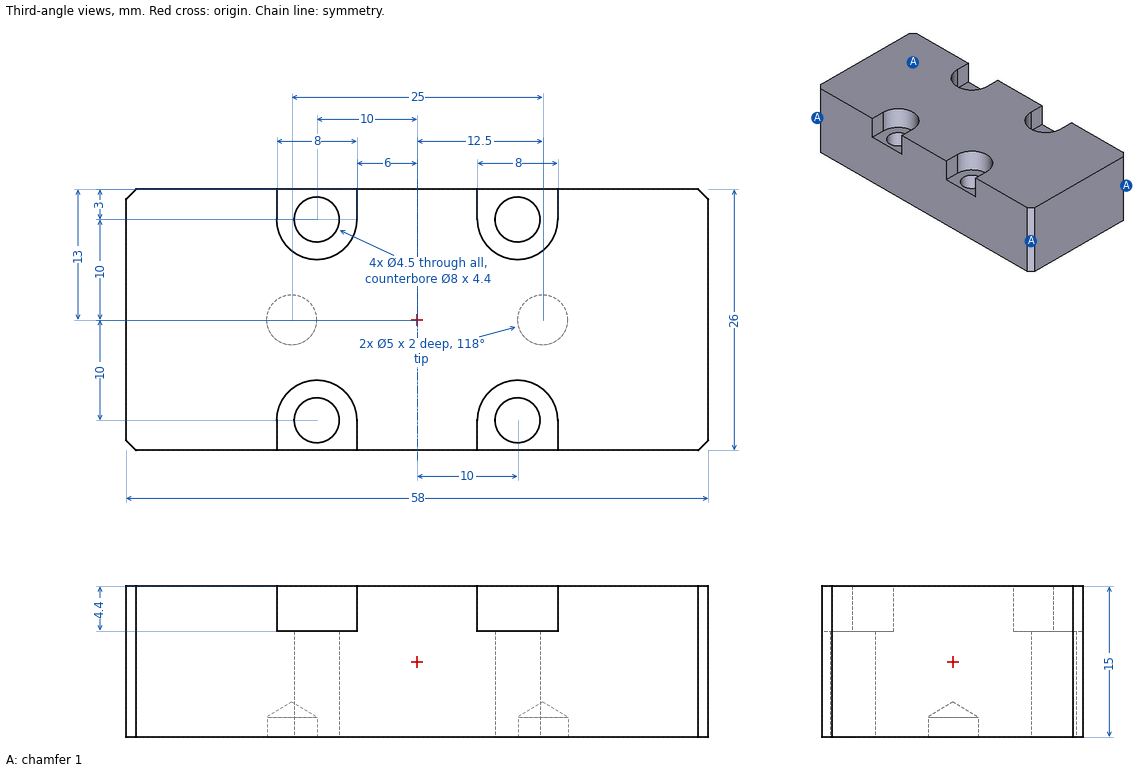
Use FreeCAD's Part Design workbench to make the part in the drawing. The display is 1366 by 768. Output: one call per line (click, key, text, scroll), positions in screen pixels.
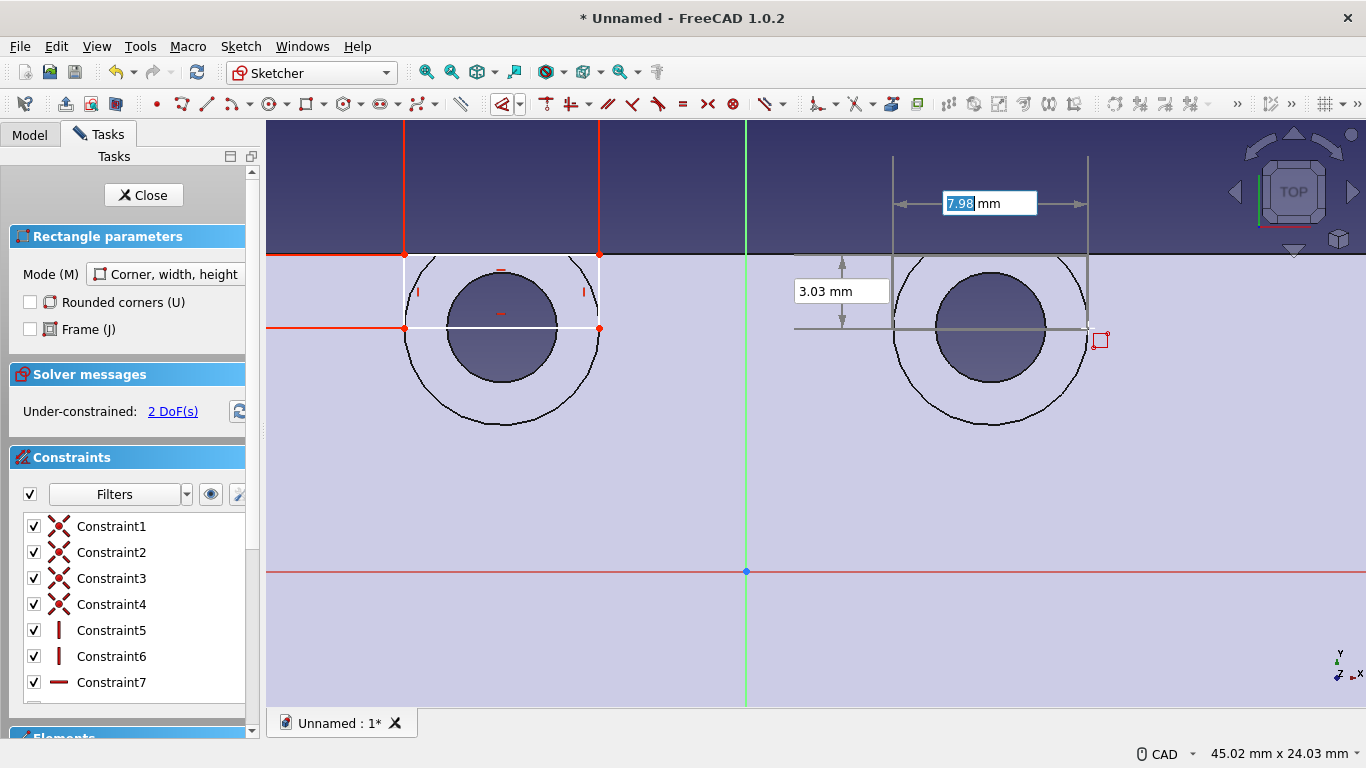
text(8)
key(Tab)
text(3)
key(Return)
key(Escape)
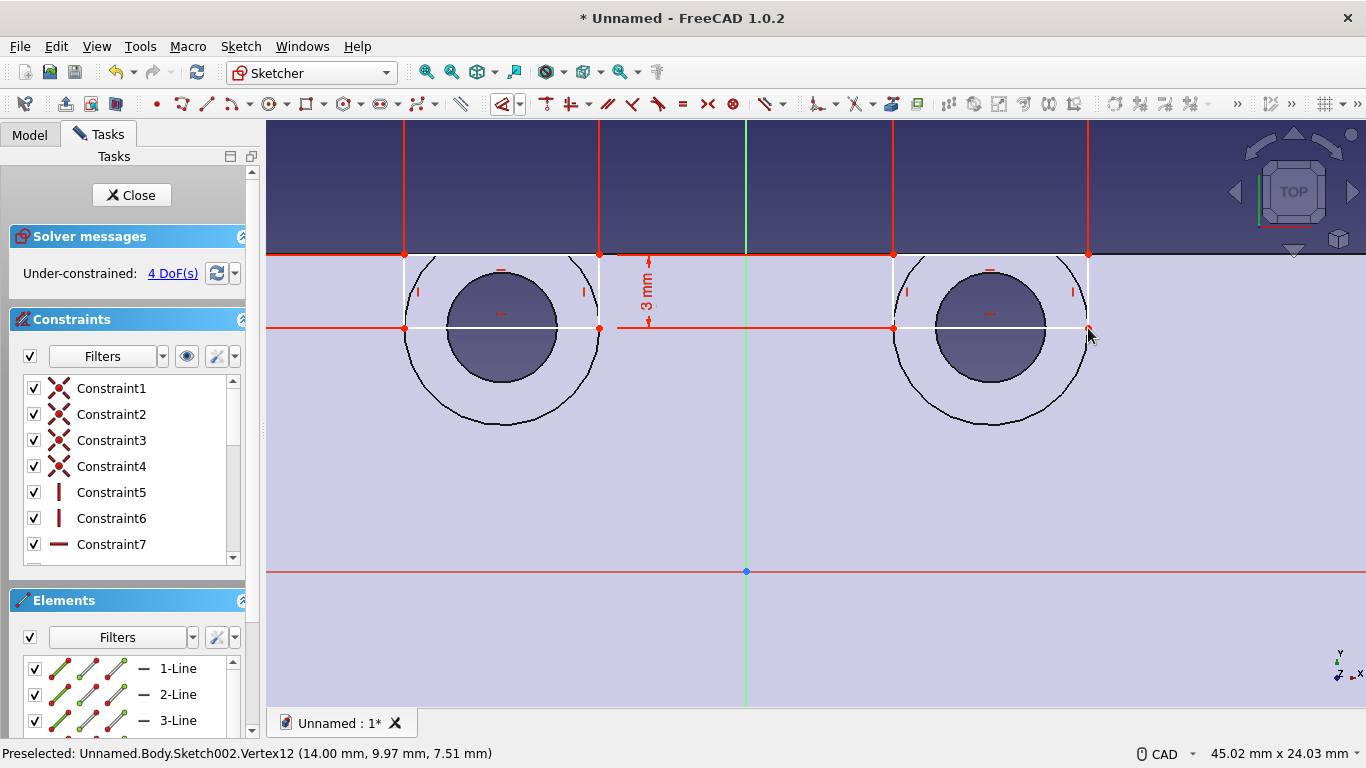
click(599, 255)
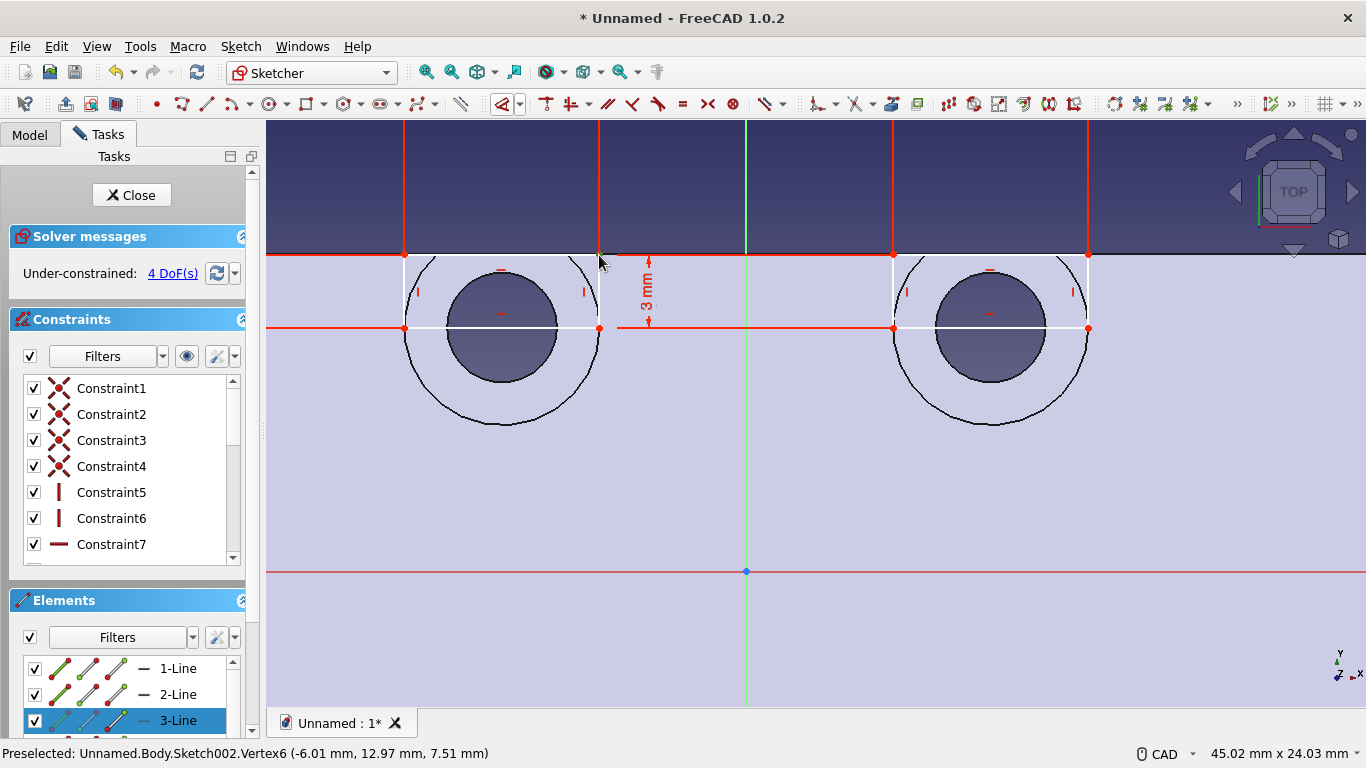
click(893, 255)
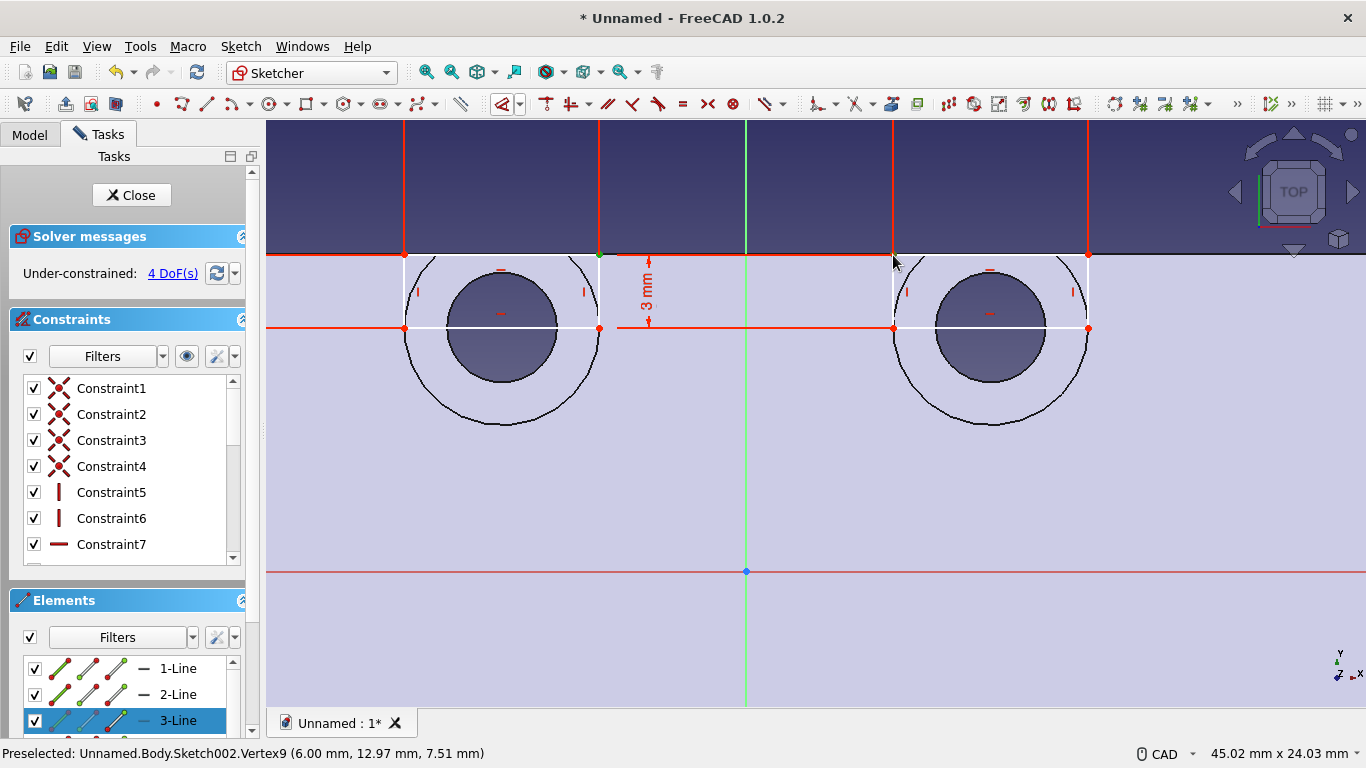
click(746, 641)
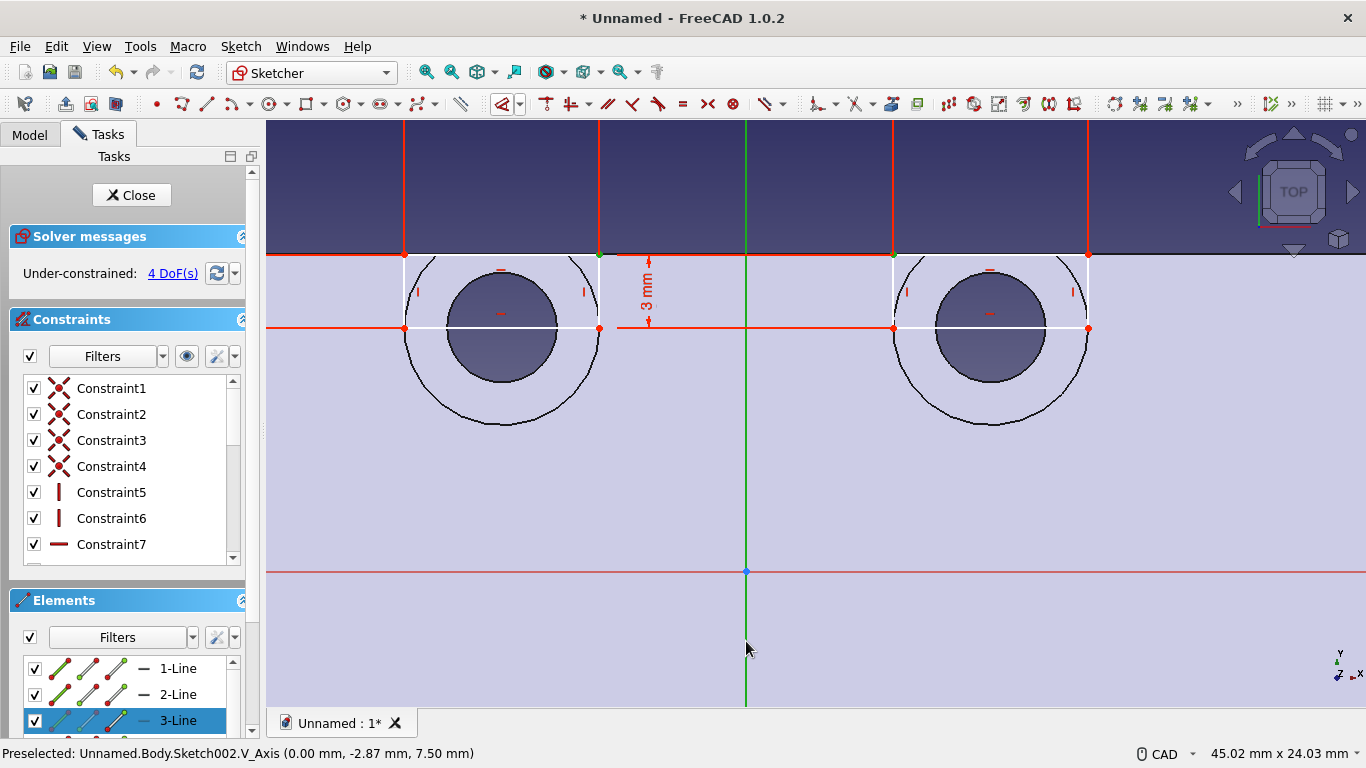
key(s)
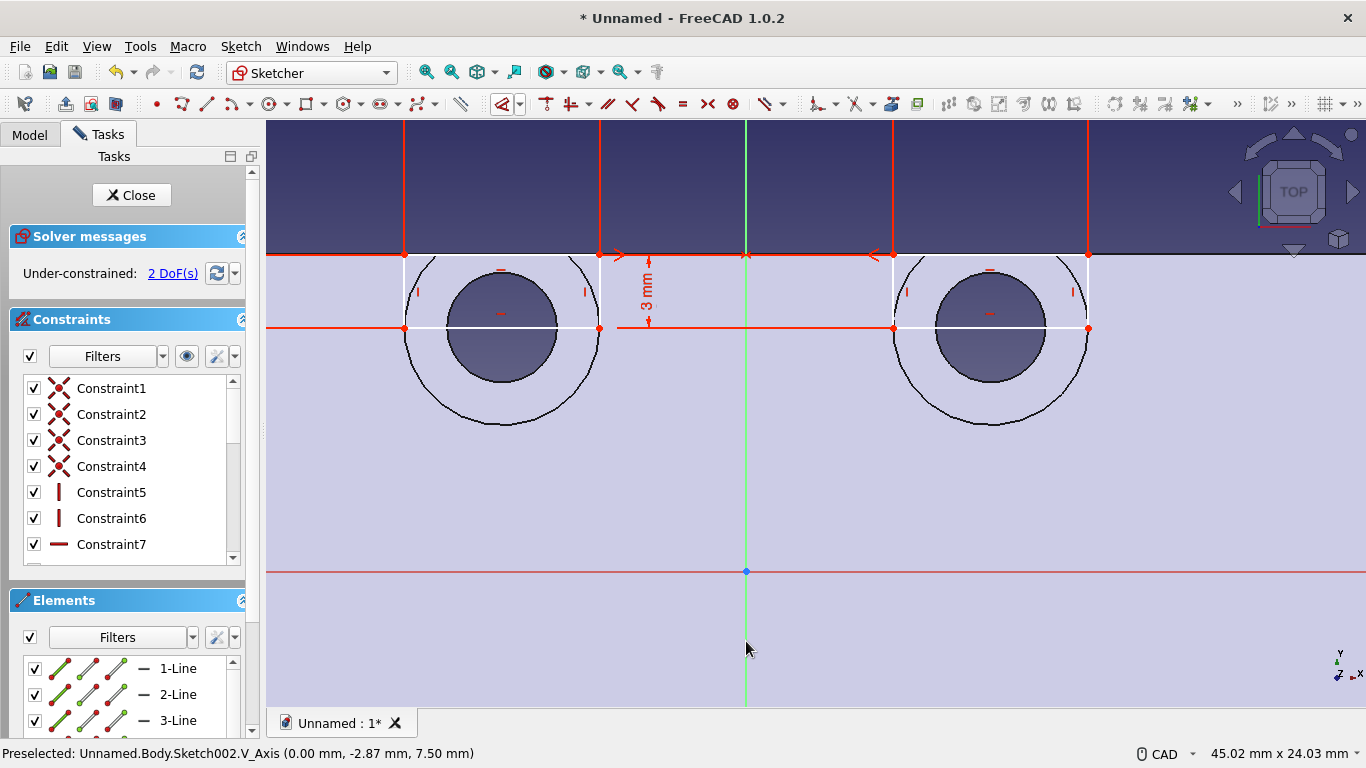
click(600, 328)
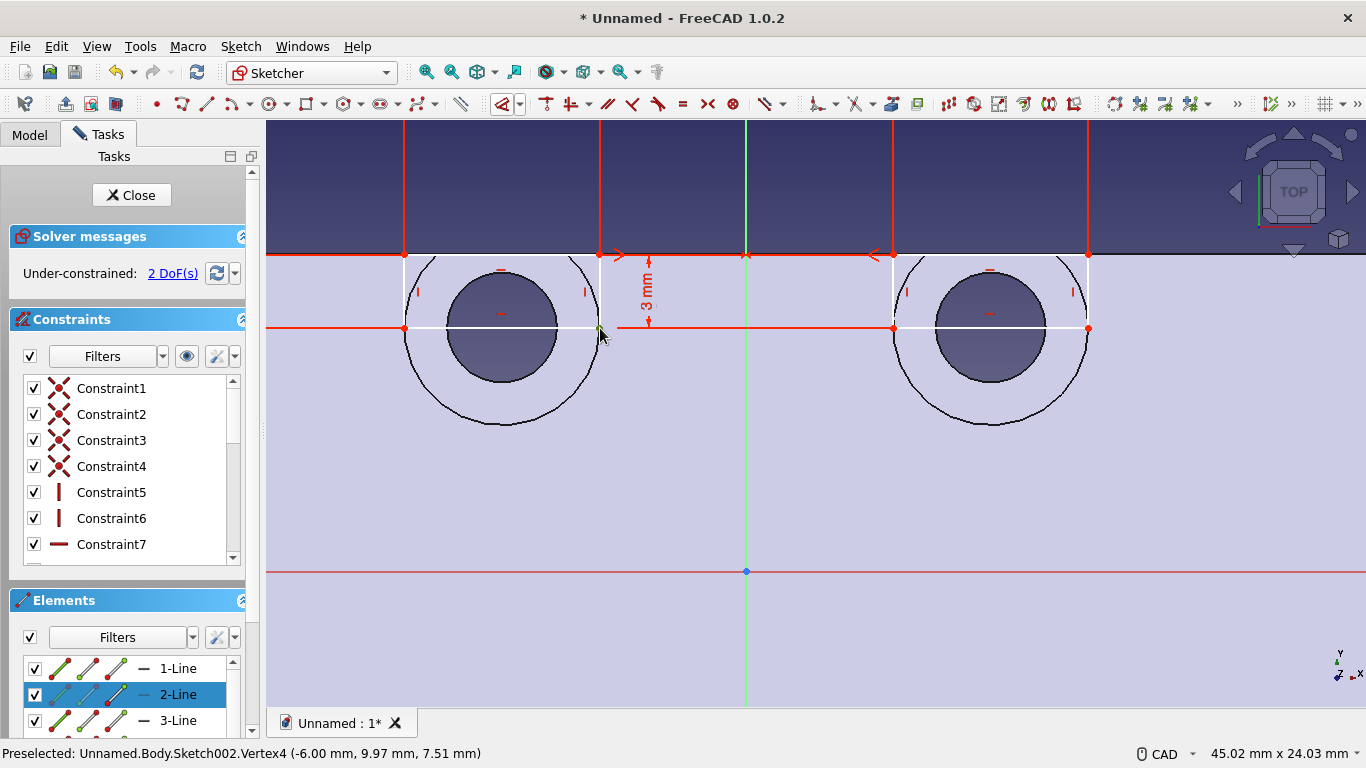
key(l)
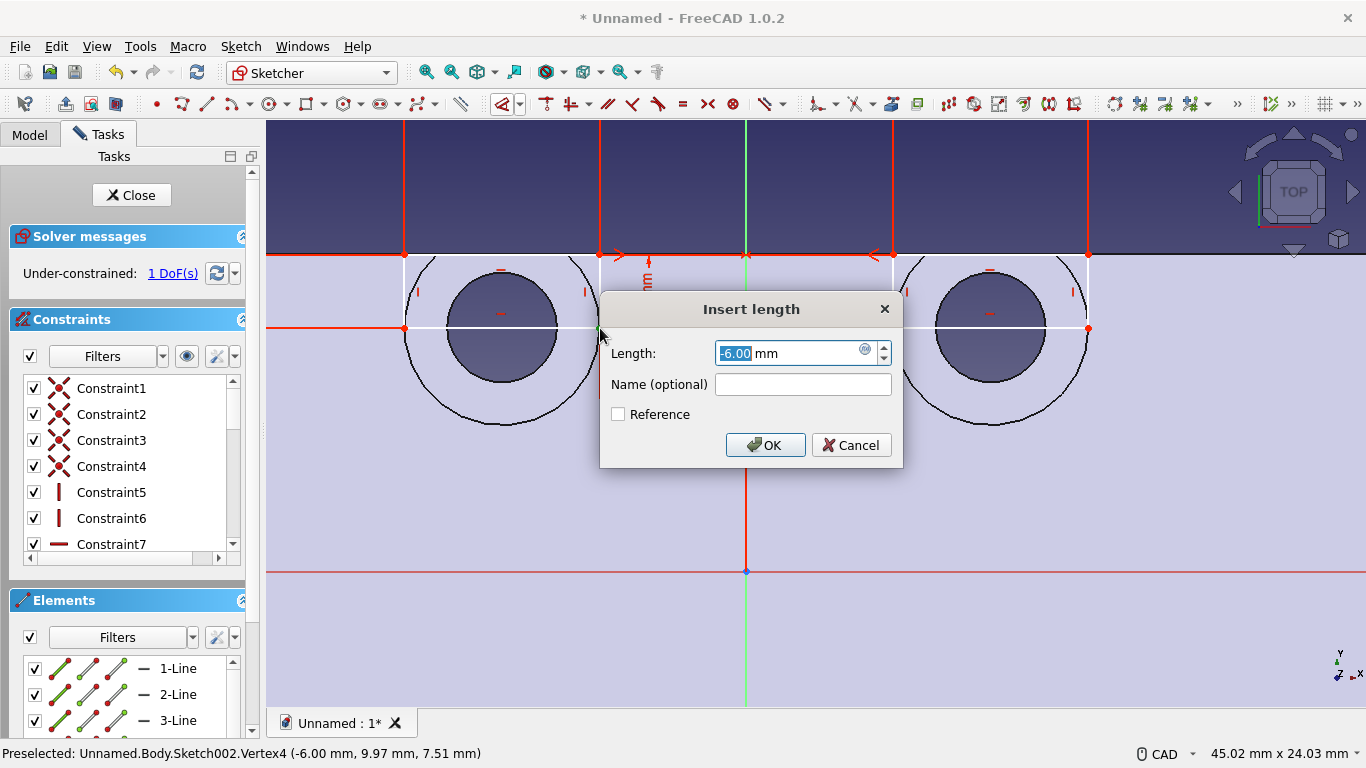
text(-6)
key(Return)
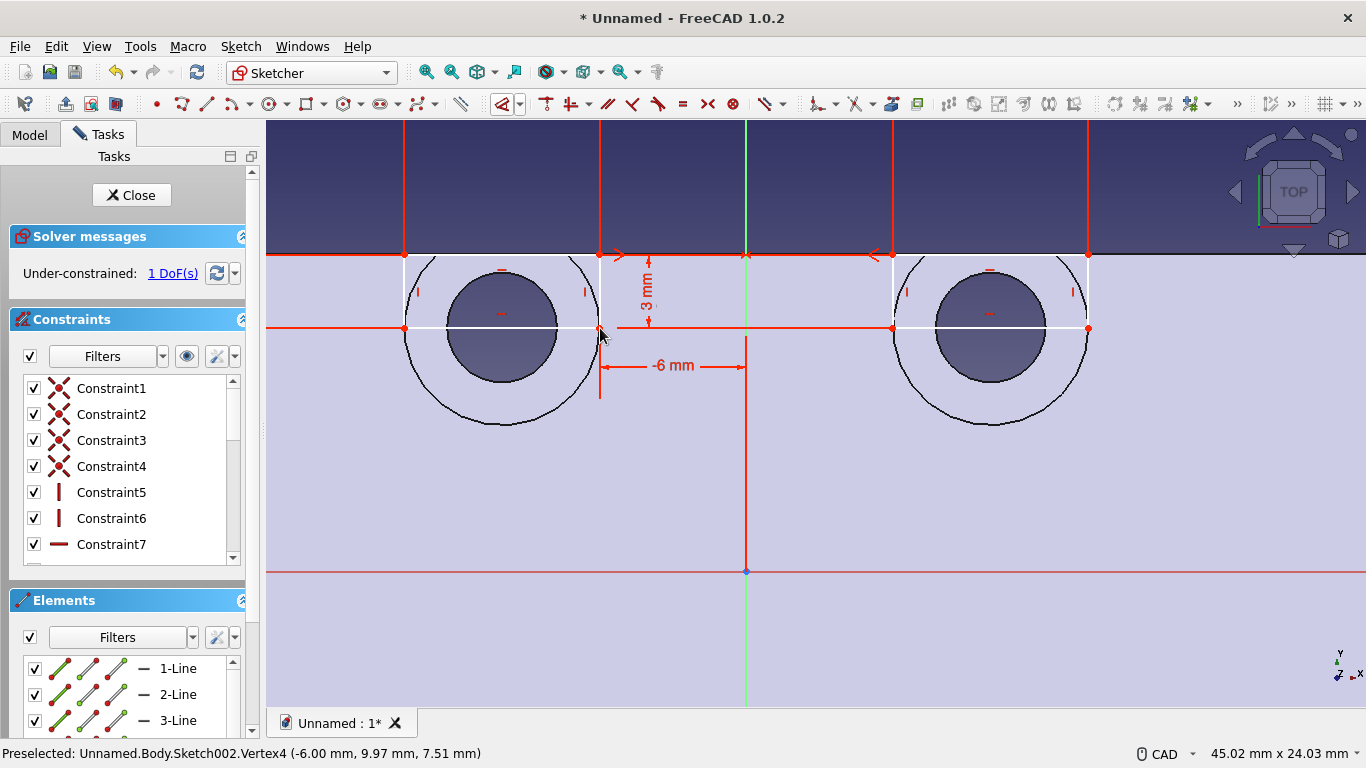
click(404, 255)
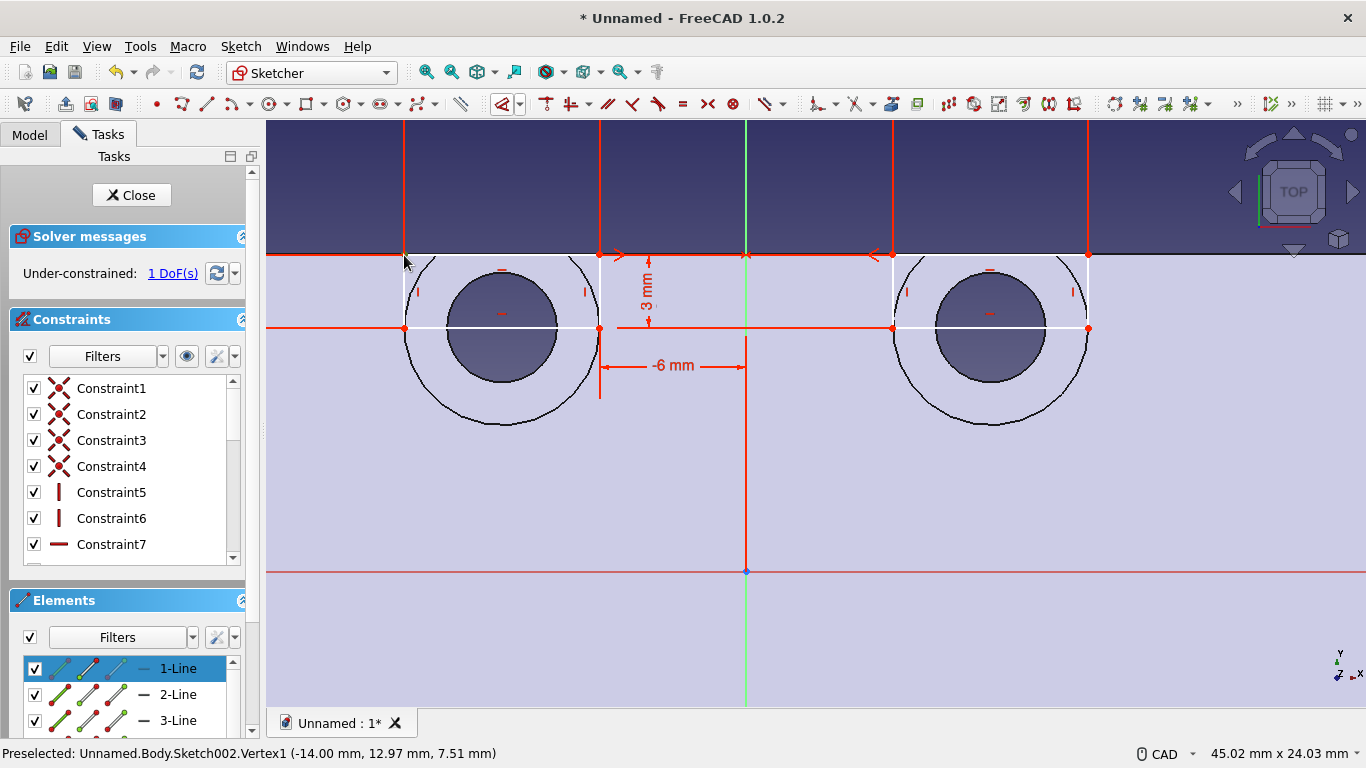
key(i)